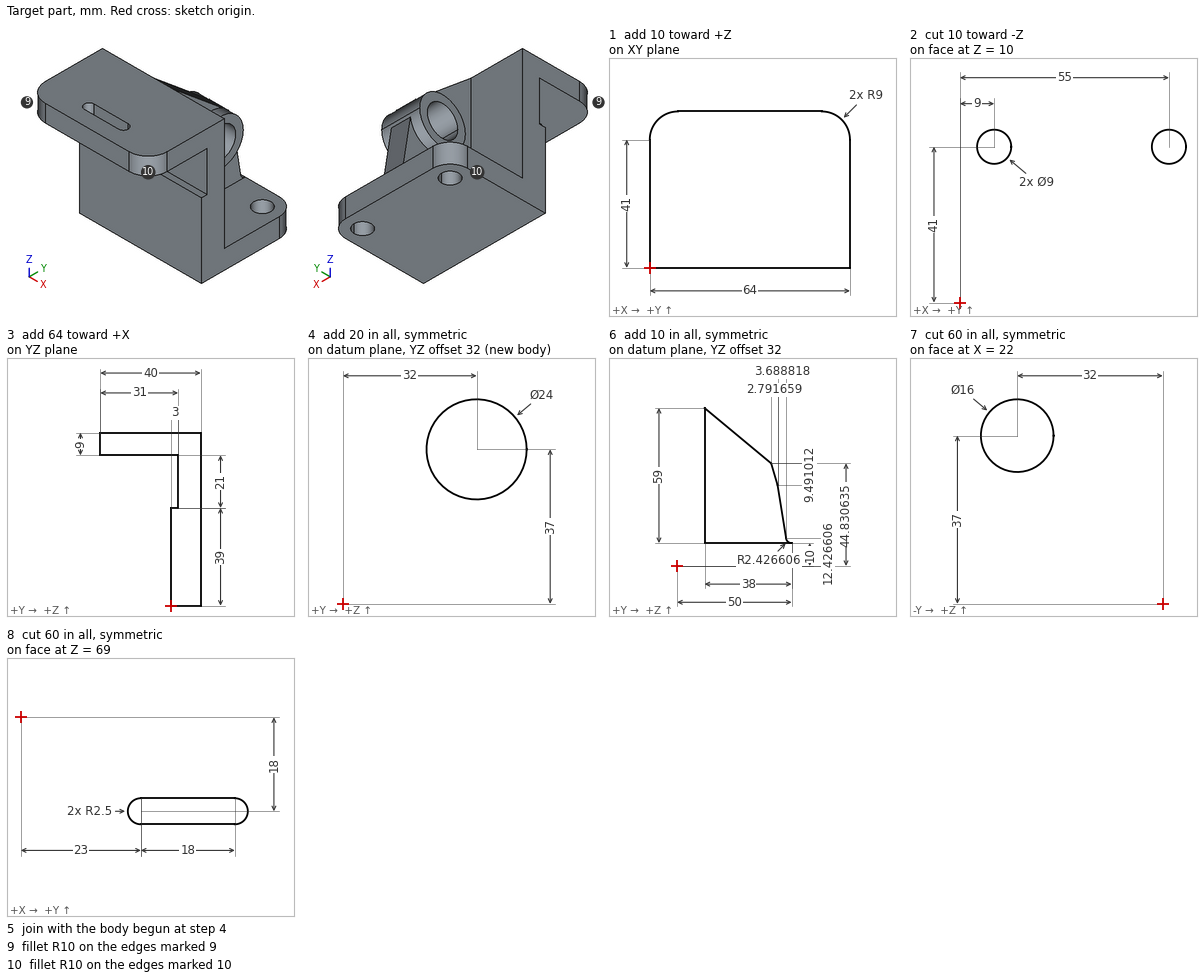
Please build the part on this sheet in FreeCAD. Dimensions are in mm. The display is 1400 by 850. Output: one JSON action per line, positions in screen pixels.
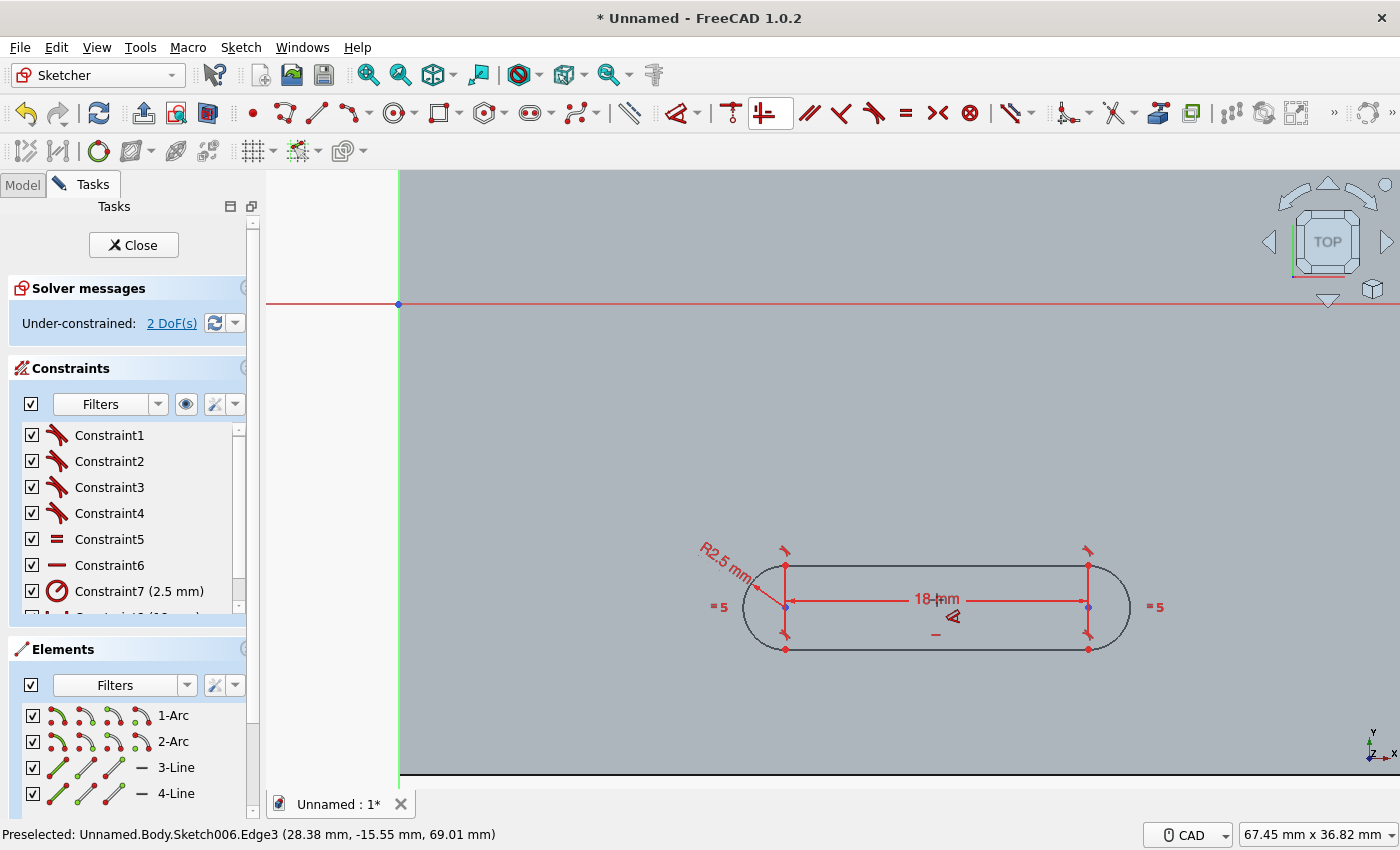
{"action": "left_click", "coordinate": [785, 566]}
{"action": "left_click", "coordinate": [592, 270]}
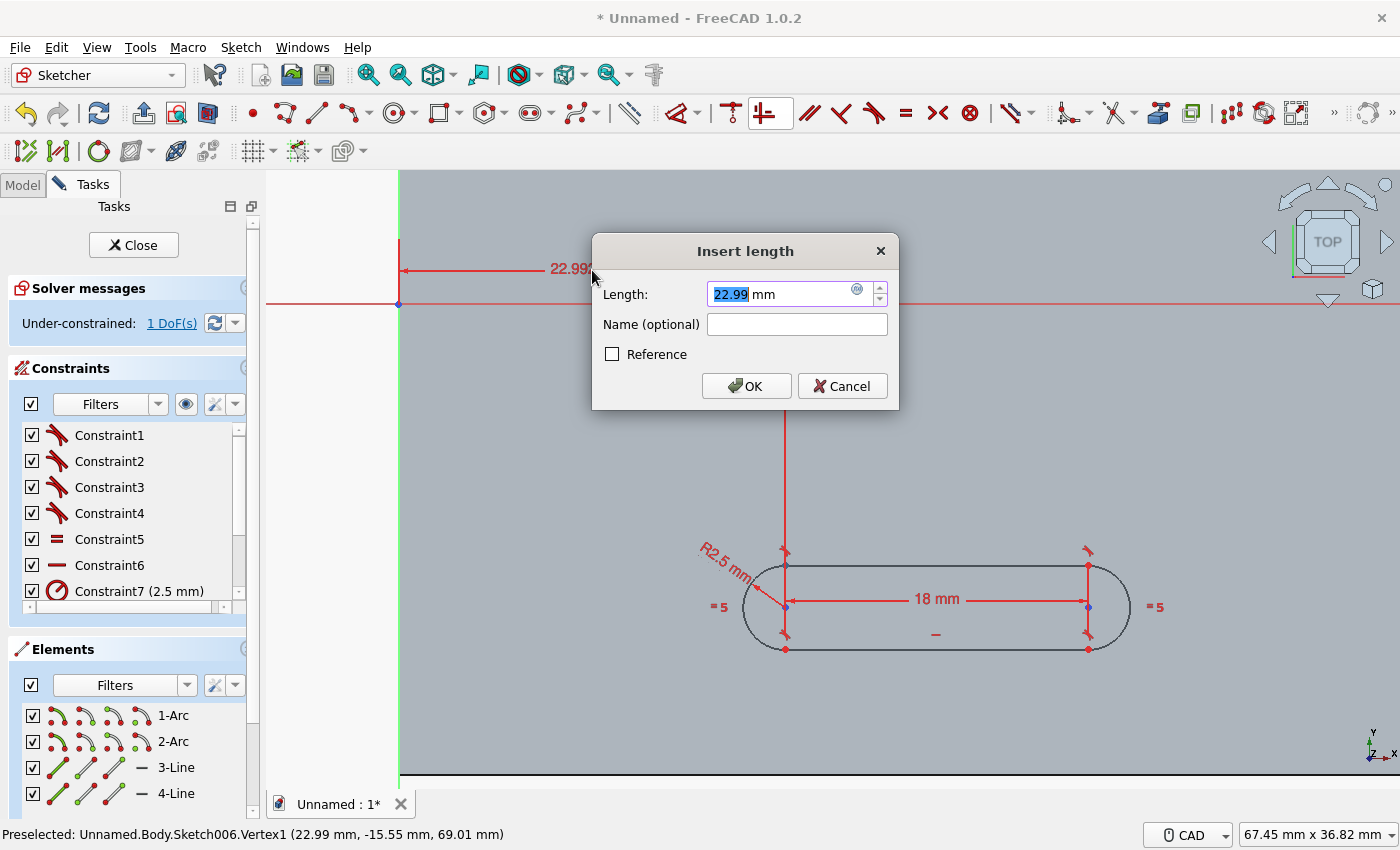
{"action": "type", "text": "23"}
{"action": "key", "text": "Return"}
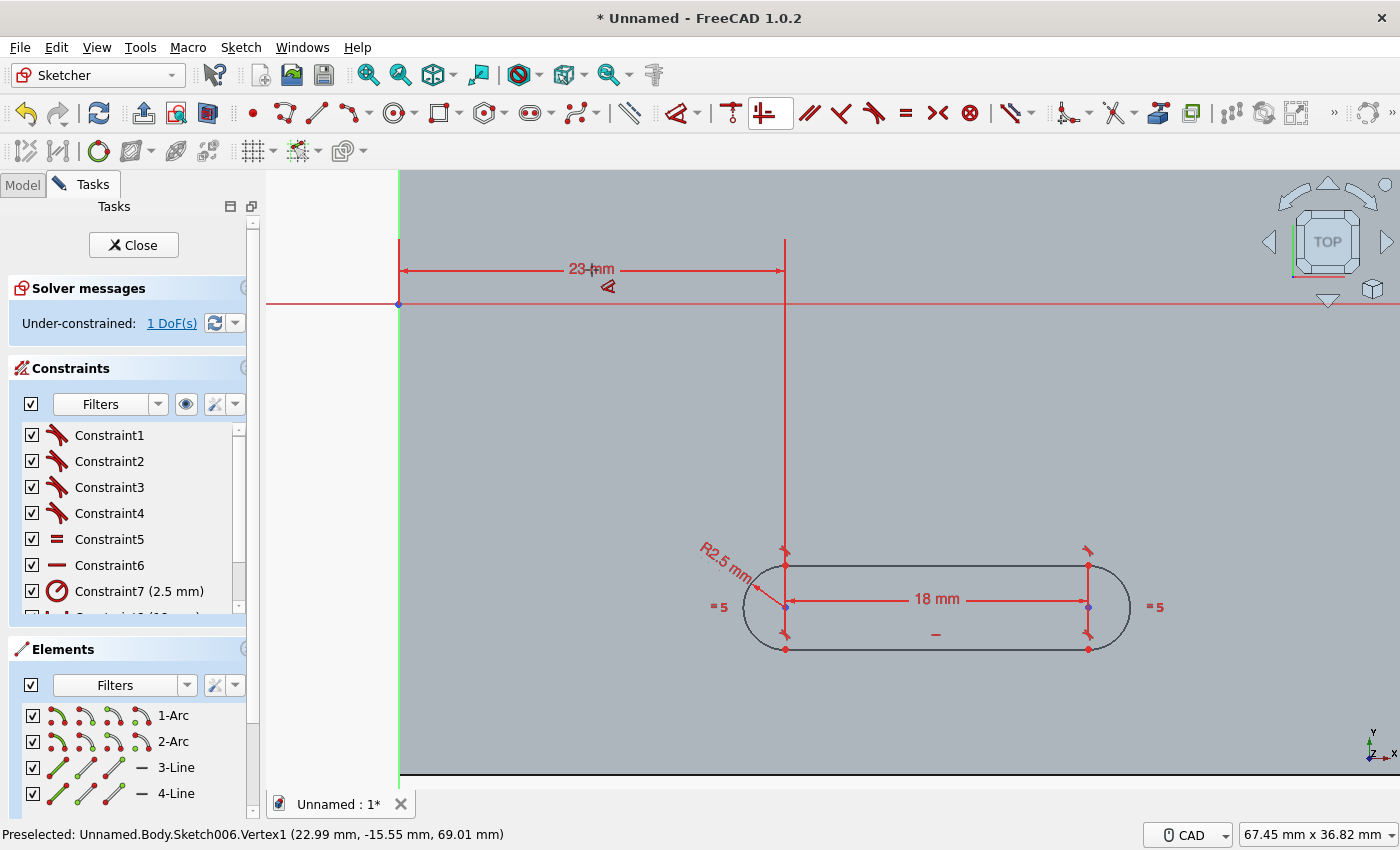
{"action": "left_click", "coordinate": [785, 608]}
{"action": "left_click", "coordinate": [365, 456]}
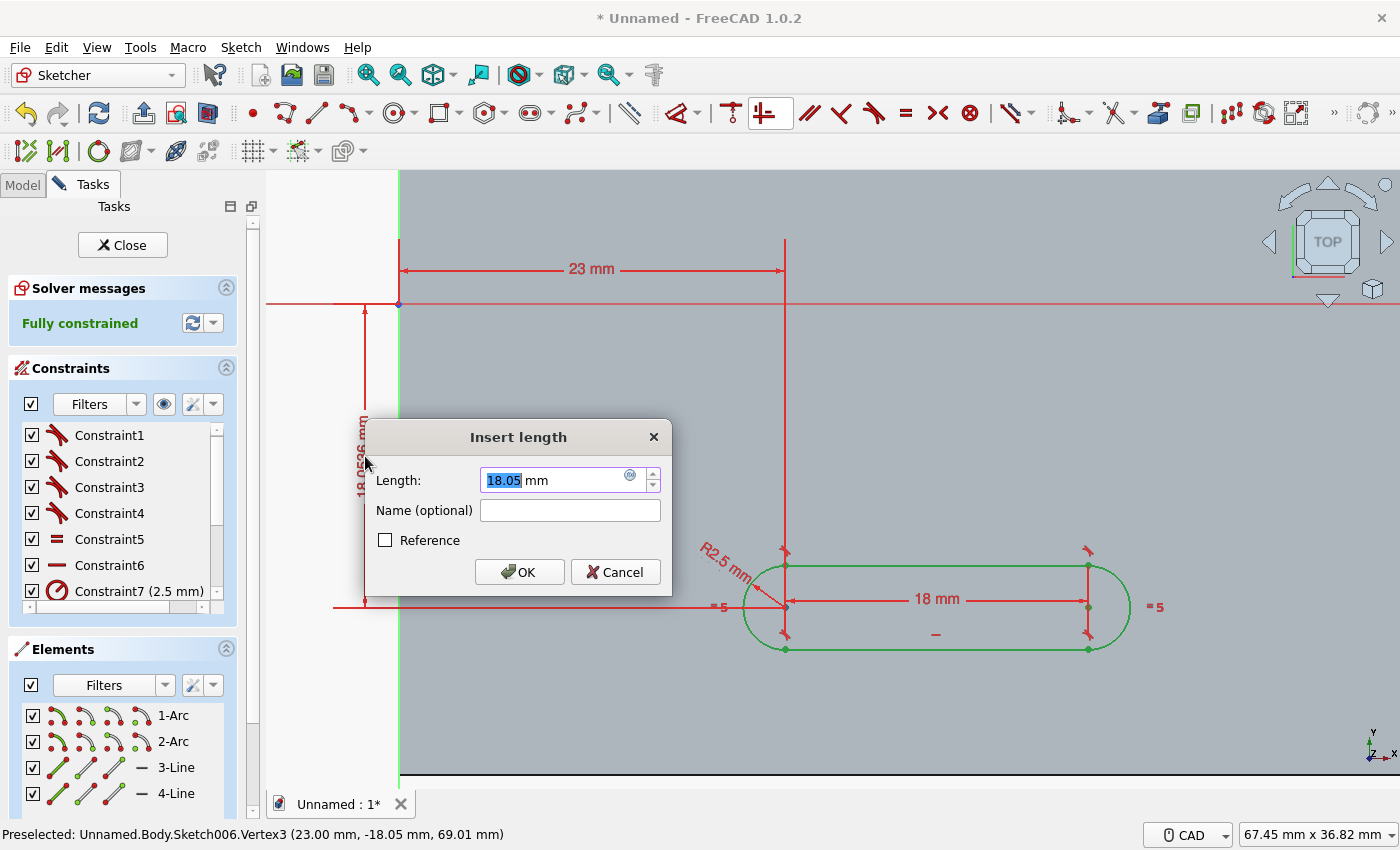
{"action": "type", "text": "18"}
{"action": "key", "text": "Return"}
{"action": "key", "text": "Escape"}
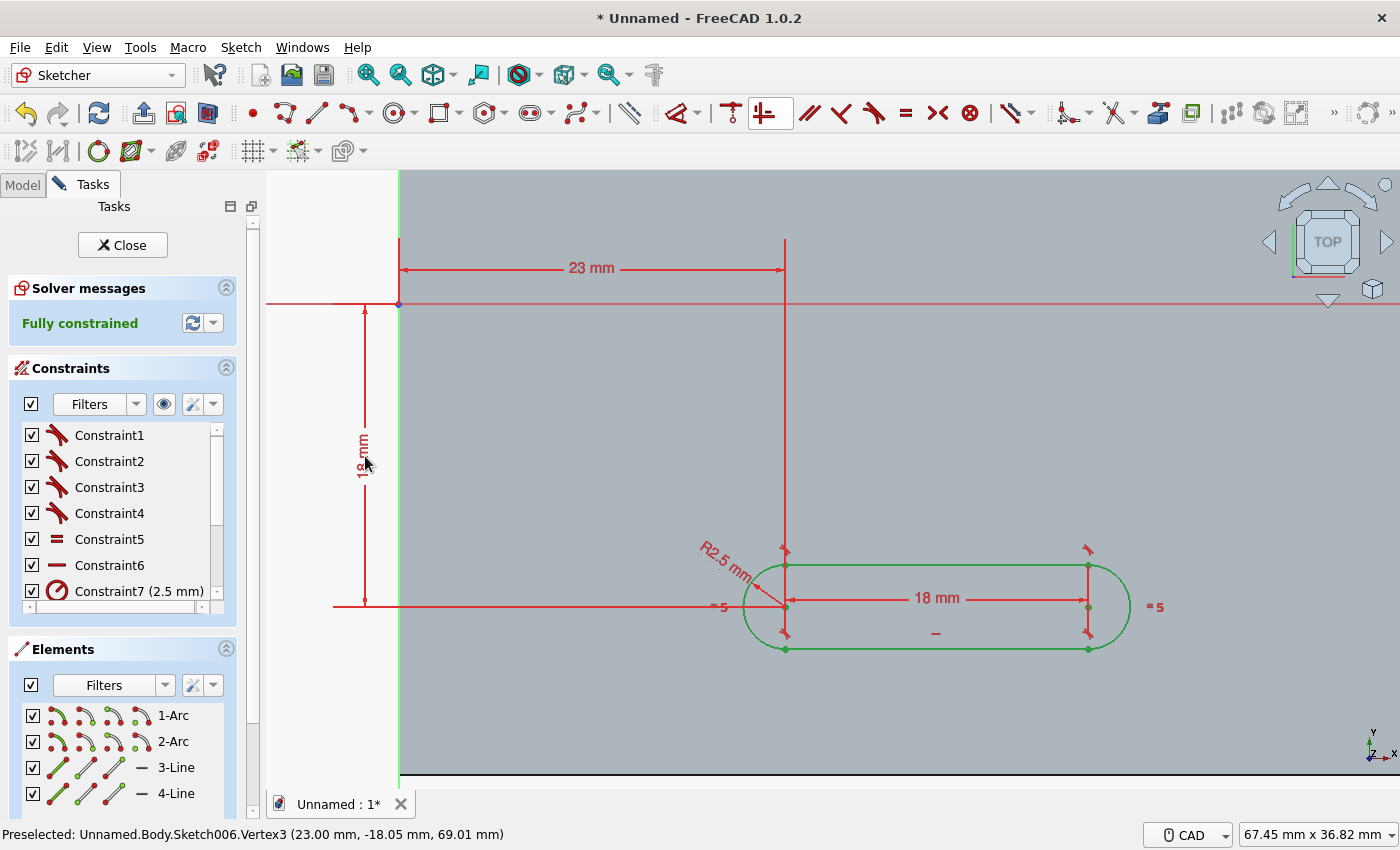
{"action": "left_click", "coordinate": [123, 245]}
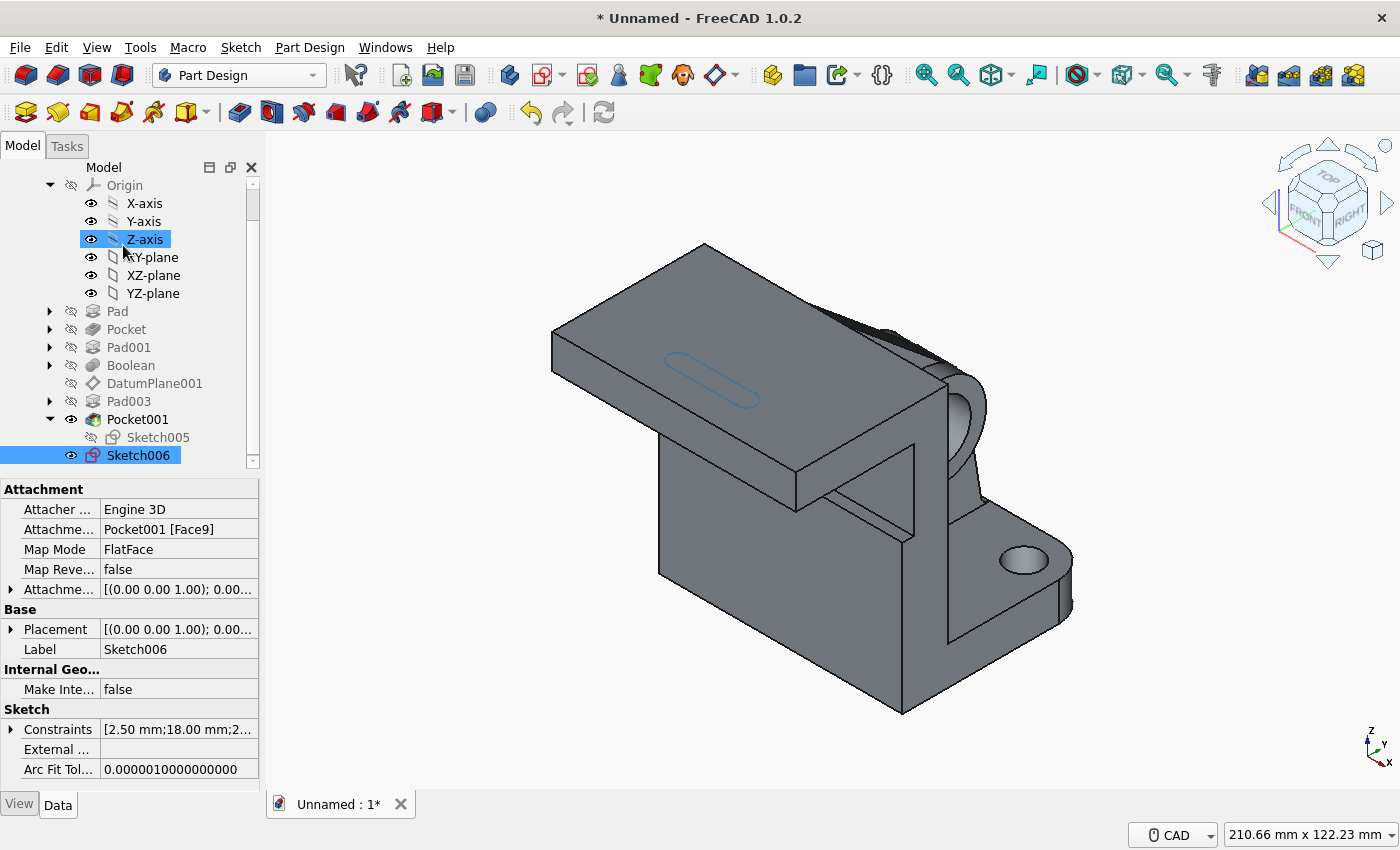
{"action": "left_click", "coordinate": [240, 112]}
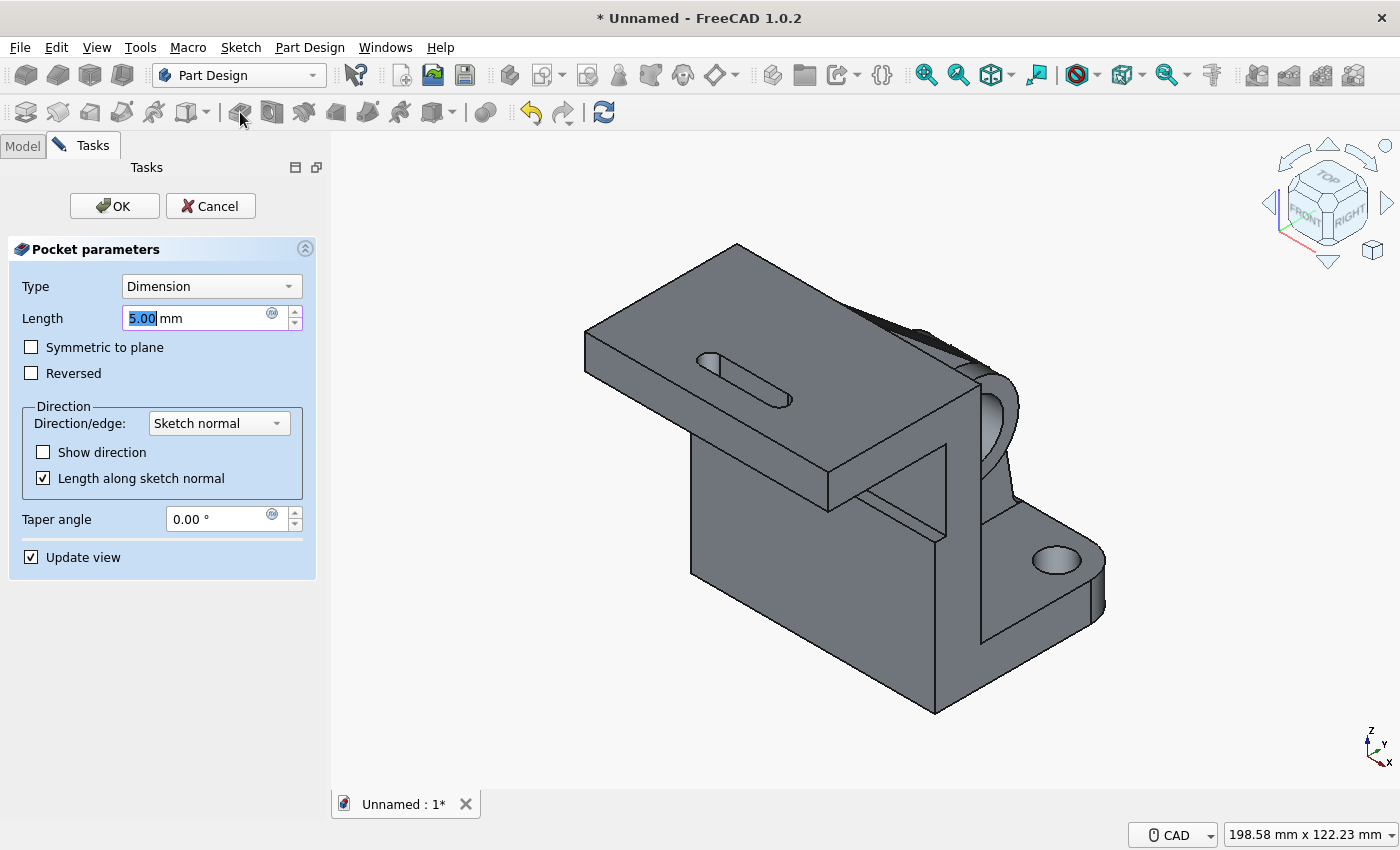
{"action": "type", "text": "60"}
{"action": "key", "text": "Tab"}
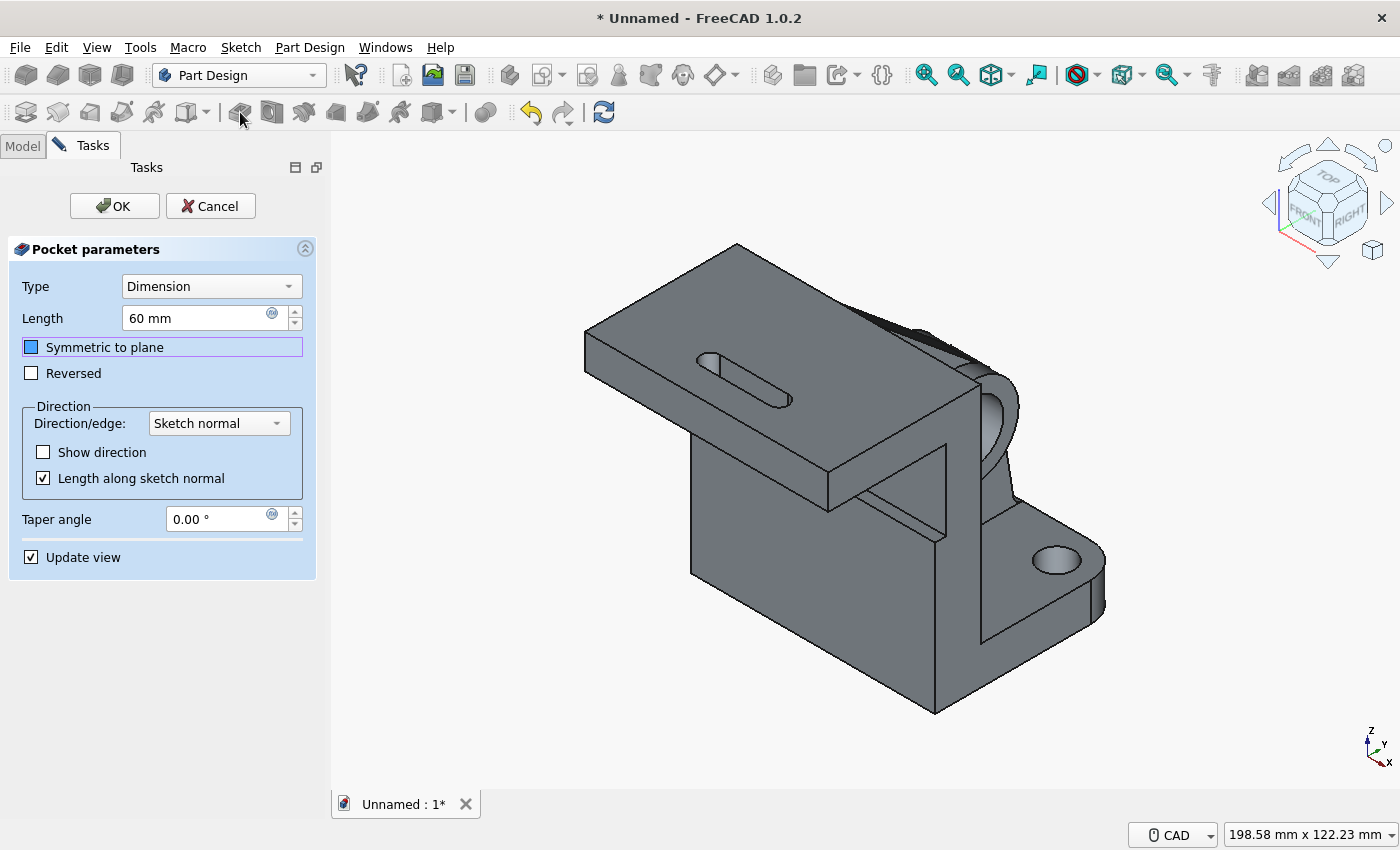
{"action": "left_click", "coordinate": [30, 347]}